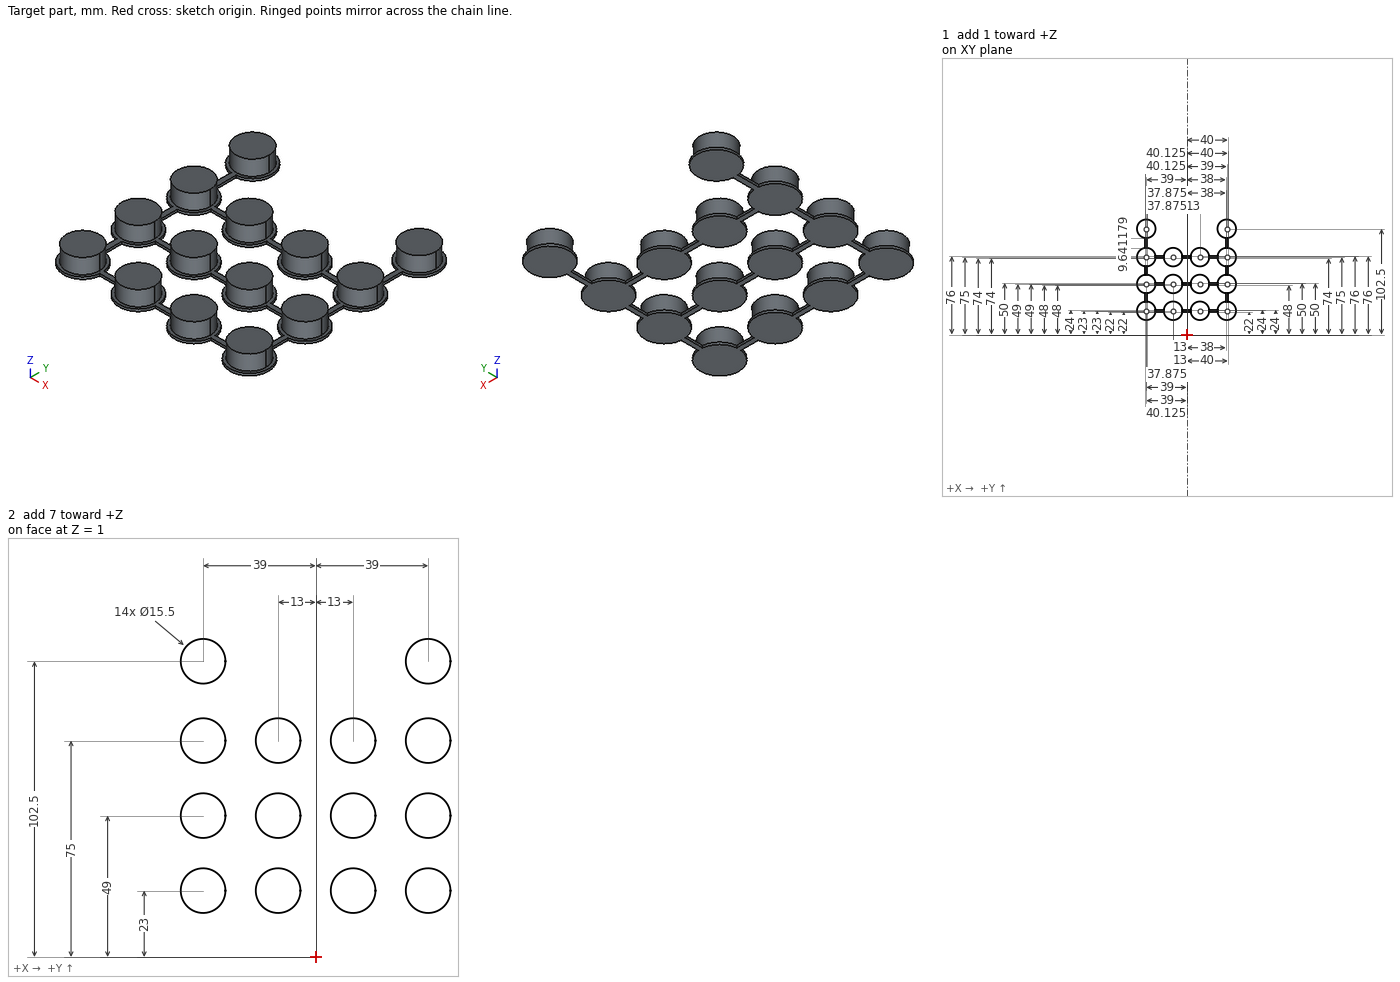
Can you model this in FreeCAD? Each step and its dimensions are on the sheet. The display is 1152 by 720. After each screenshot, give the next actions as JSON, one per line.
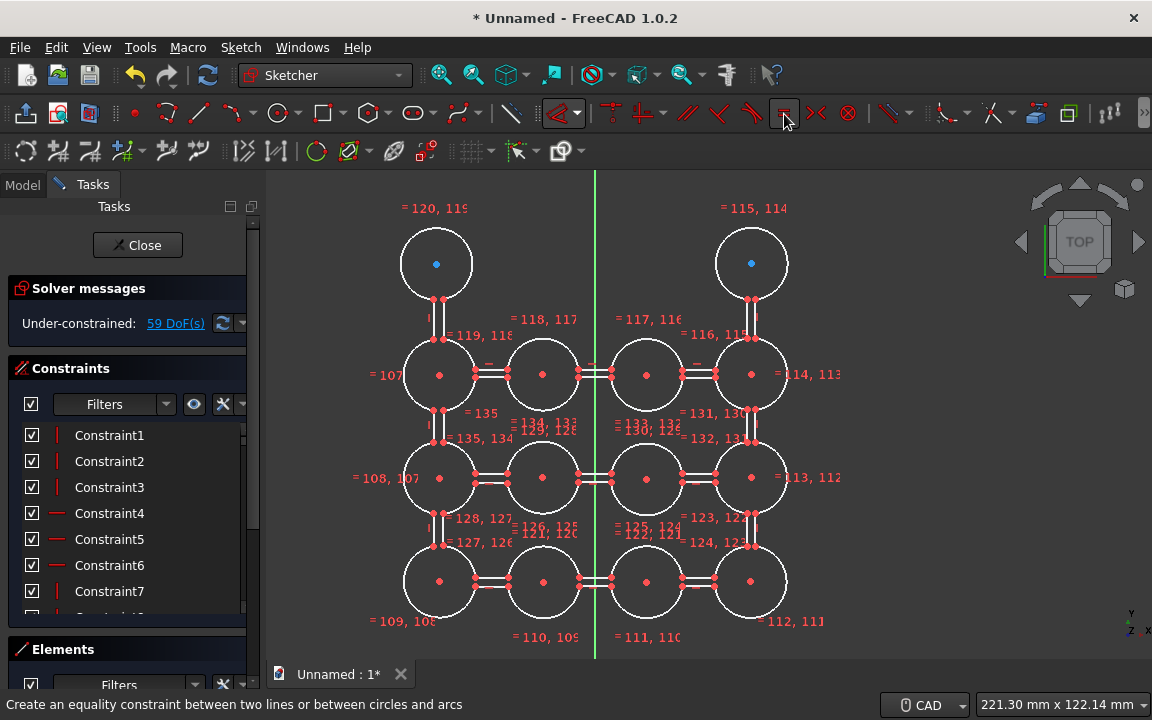
{"action": "left_click", "coordinate": [544, 582]}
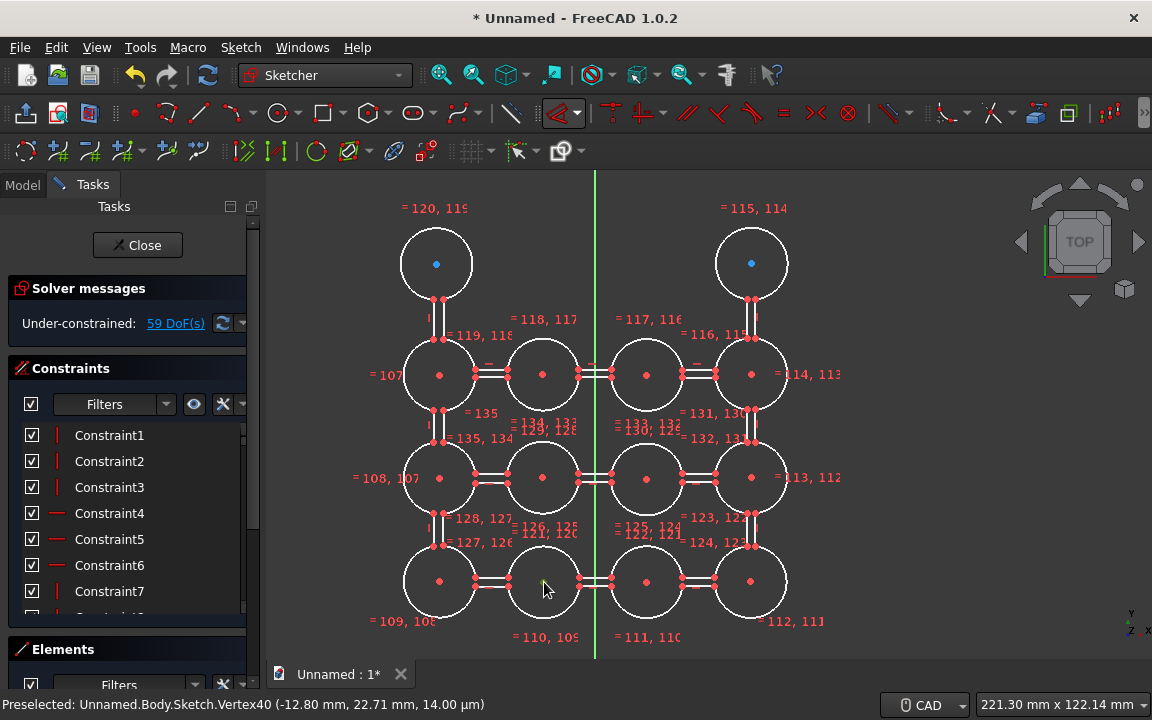
{"action": "left_click", "coordinate": [647, 582]}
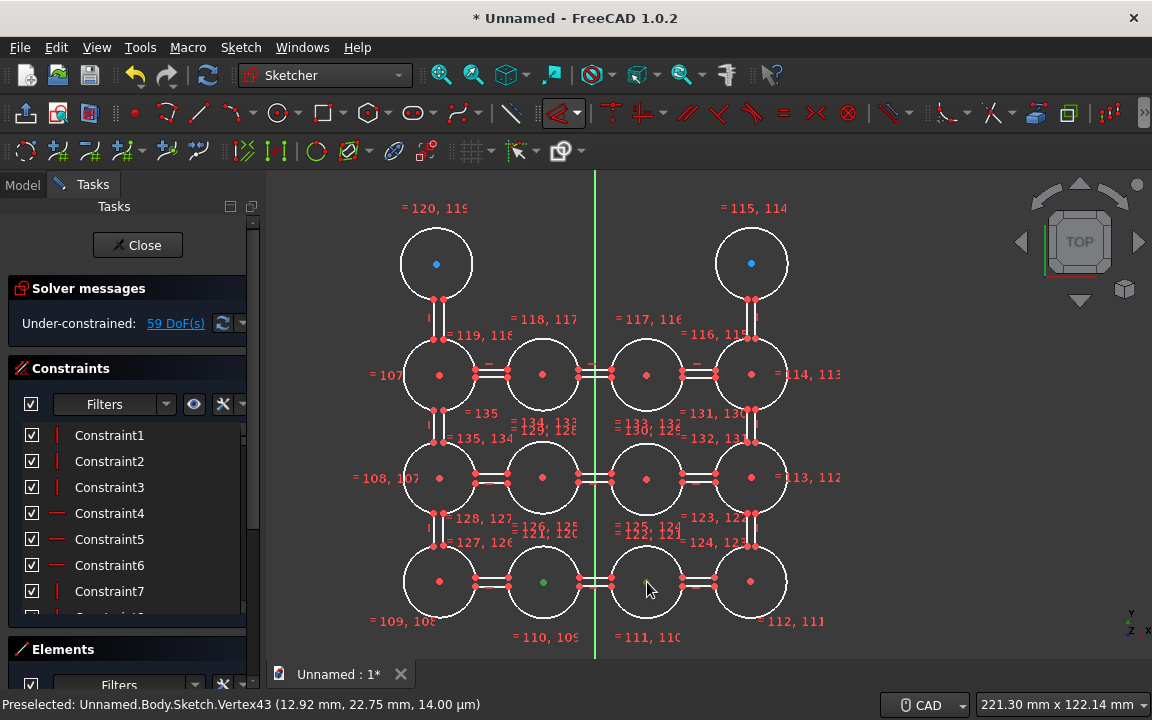
{"action": "left_click", "coordinate": [595, 538]}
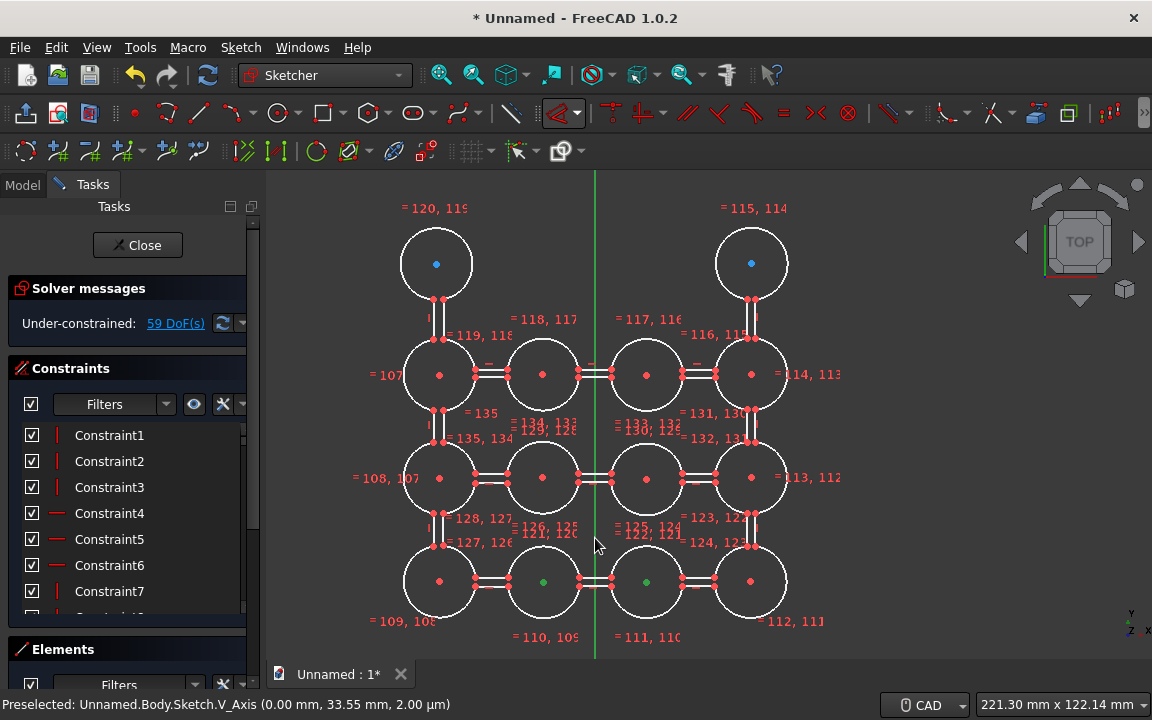
{"action": "left_click", "coordinate": [816, 114]}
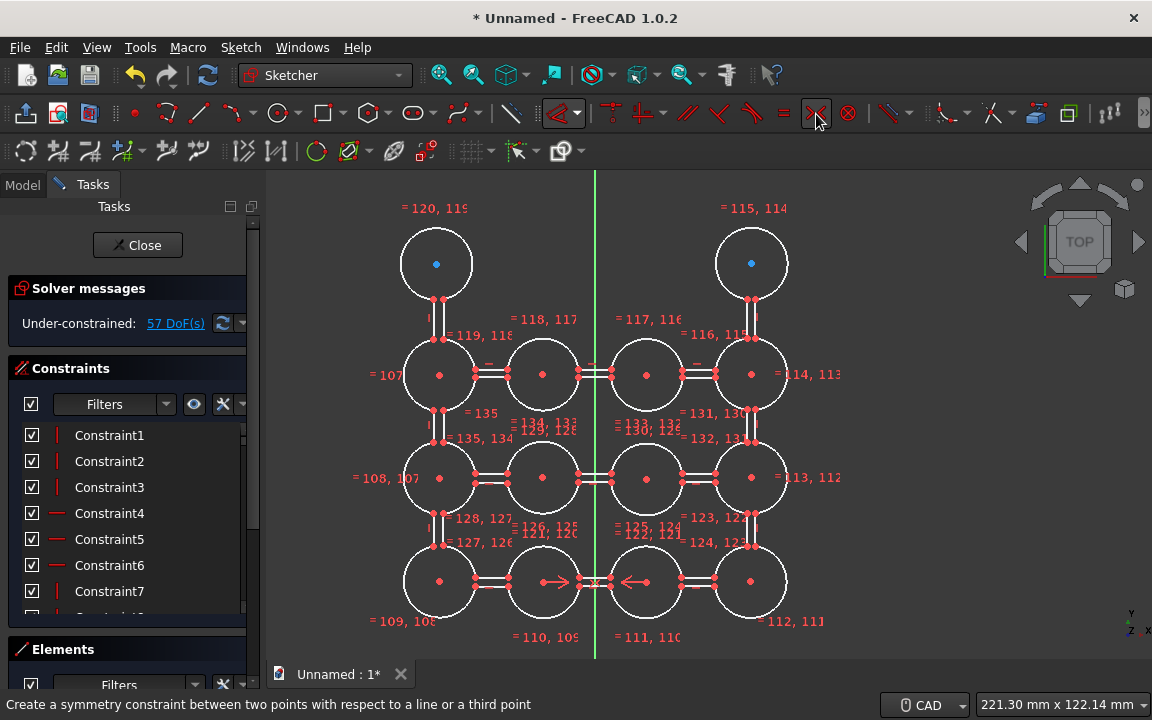
{"action": "left_click", "coordinate": [440, 582]}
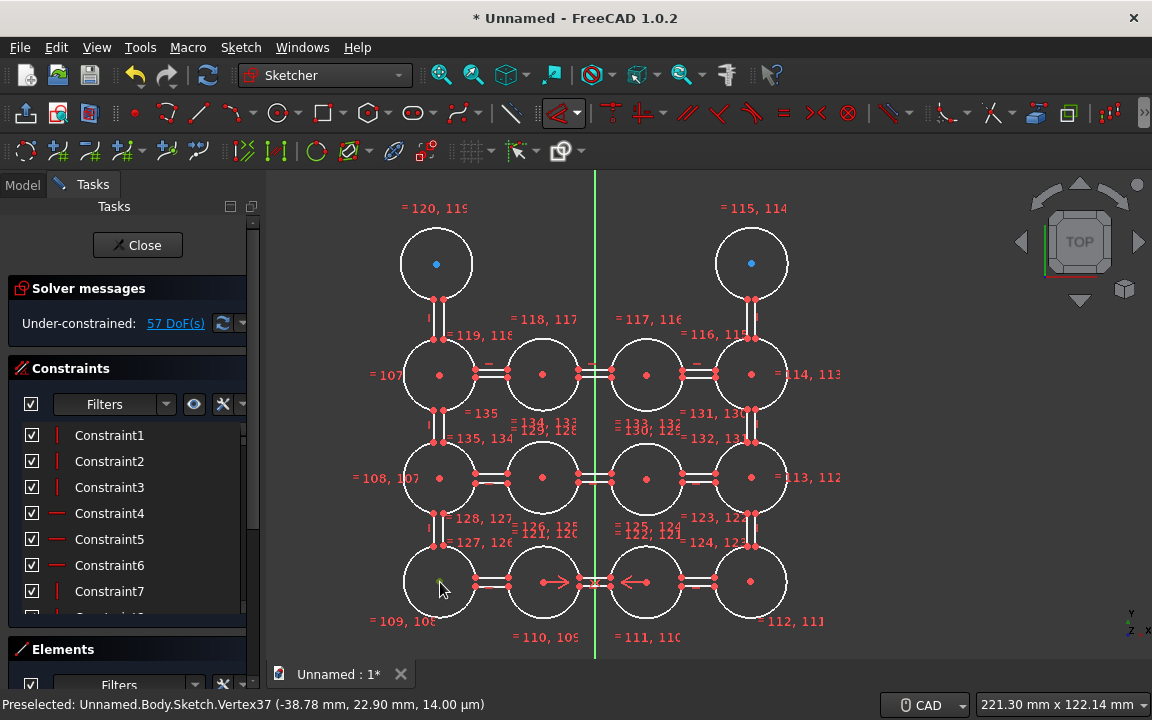
{"action": "left_click", "coordinate": [751, 582]}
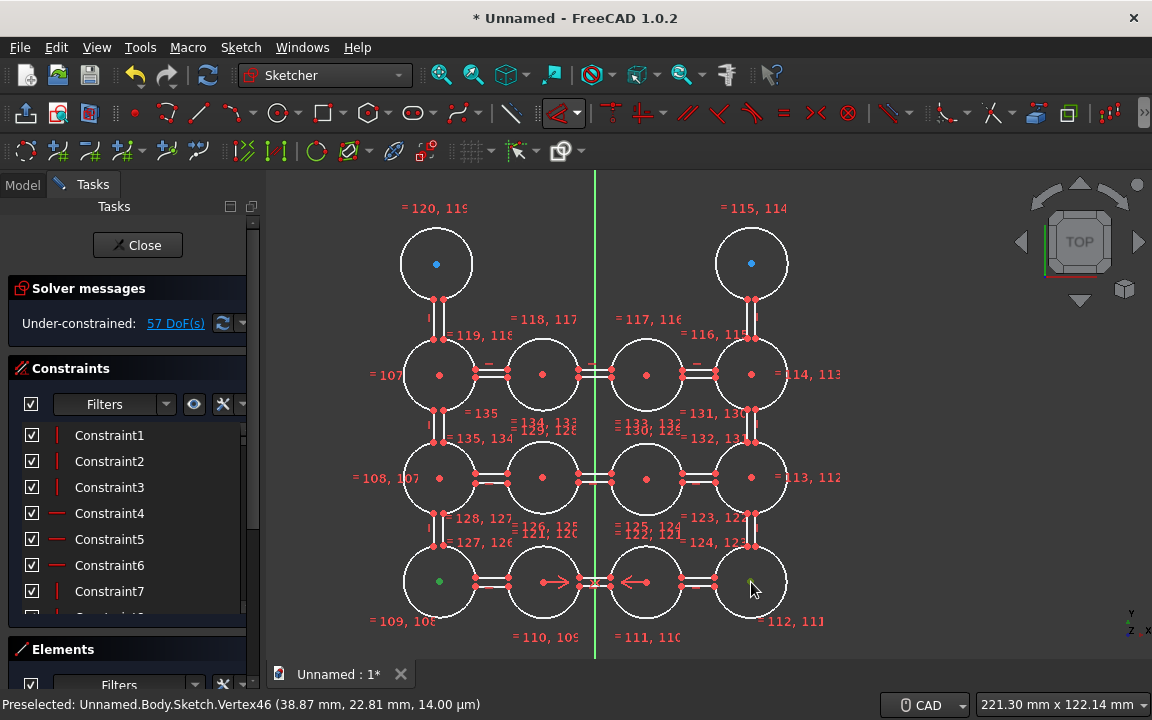
{"action": "left_click", "coordinate": [595, 538]}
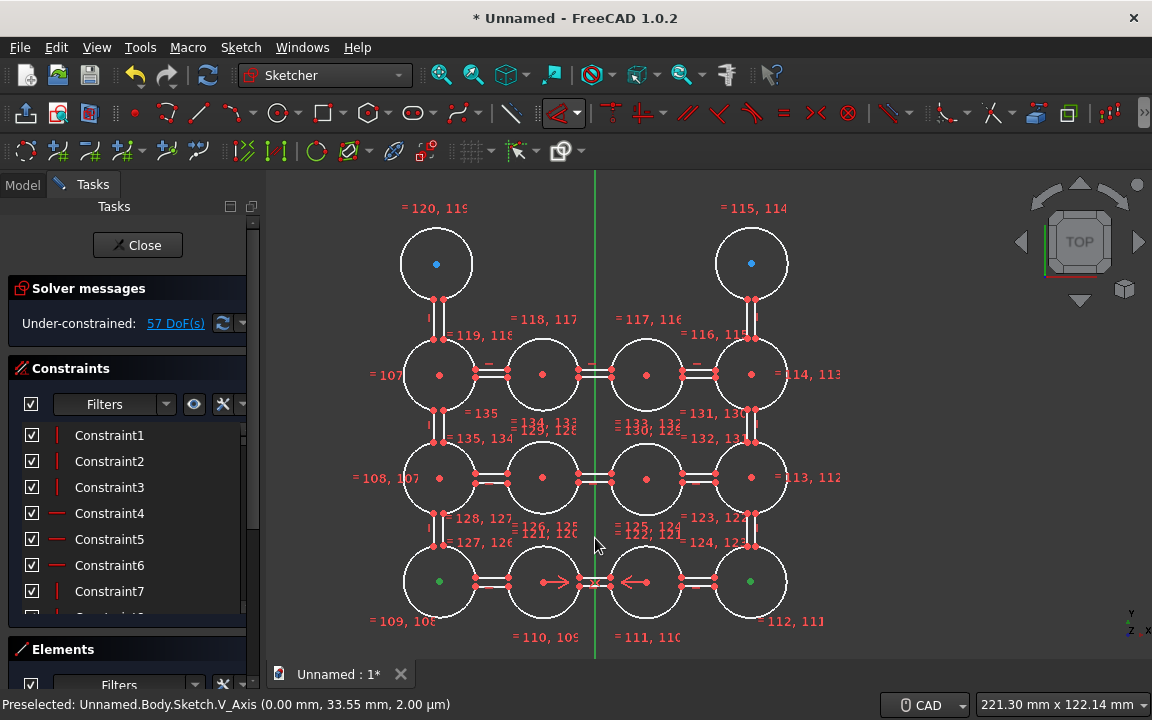
{"action": "left_click", "coordinate": [816, 114]}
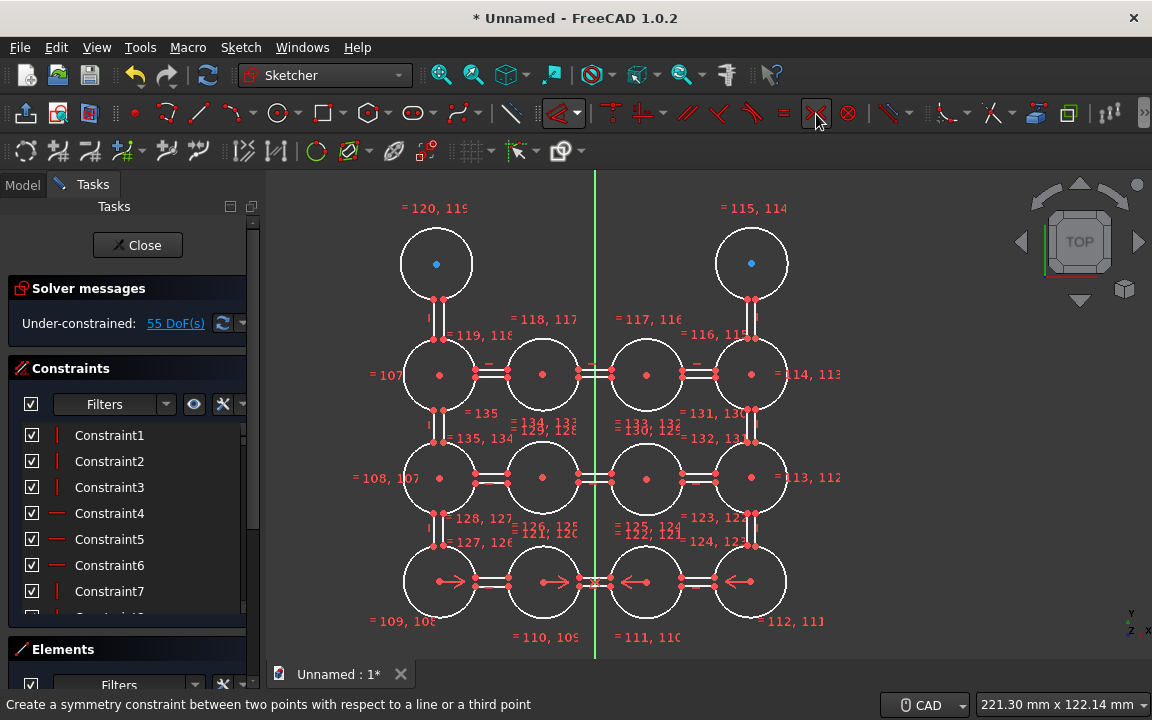
{"action": "left_click", "coordinate": [440, 478]}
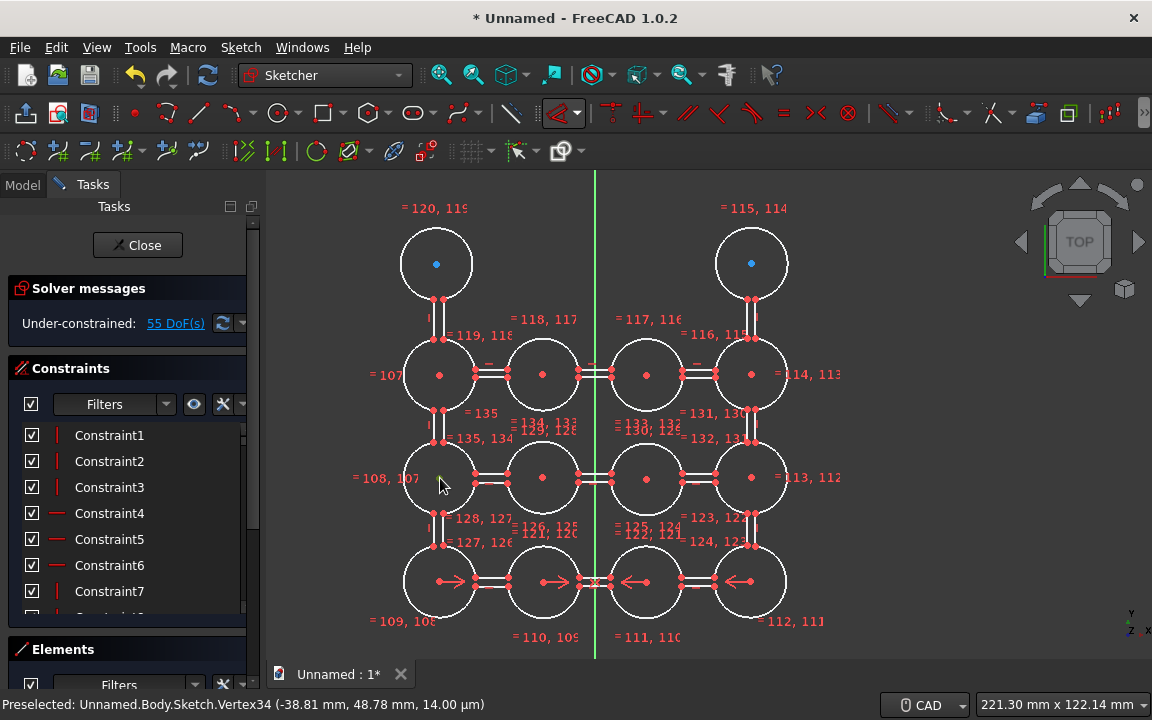
{"action": "left_click", "coordinate": [751, 478]}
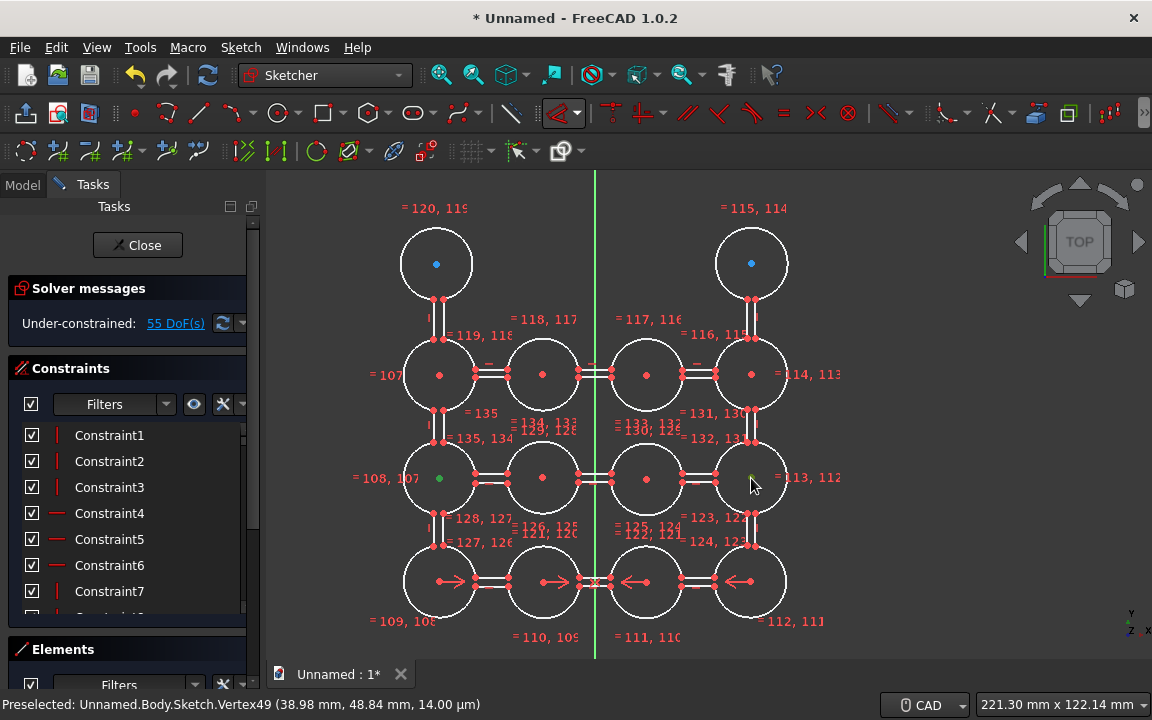
{"action": "left_click", "coordinate": [595, 538]}